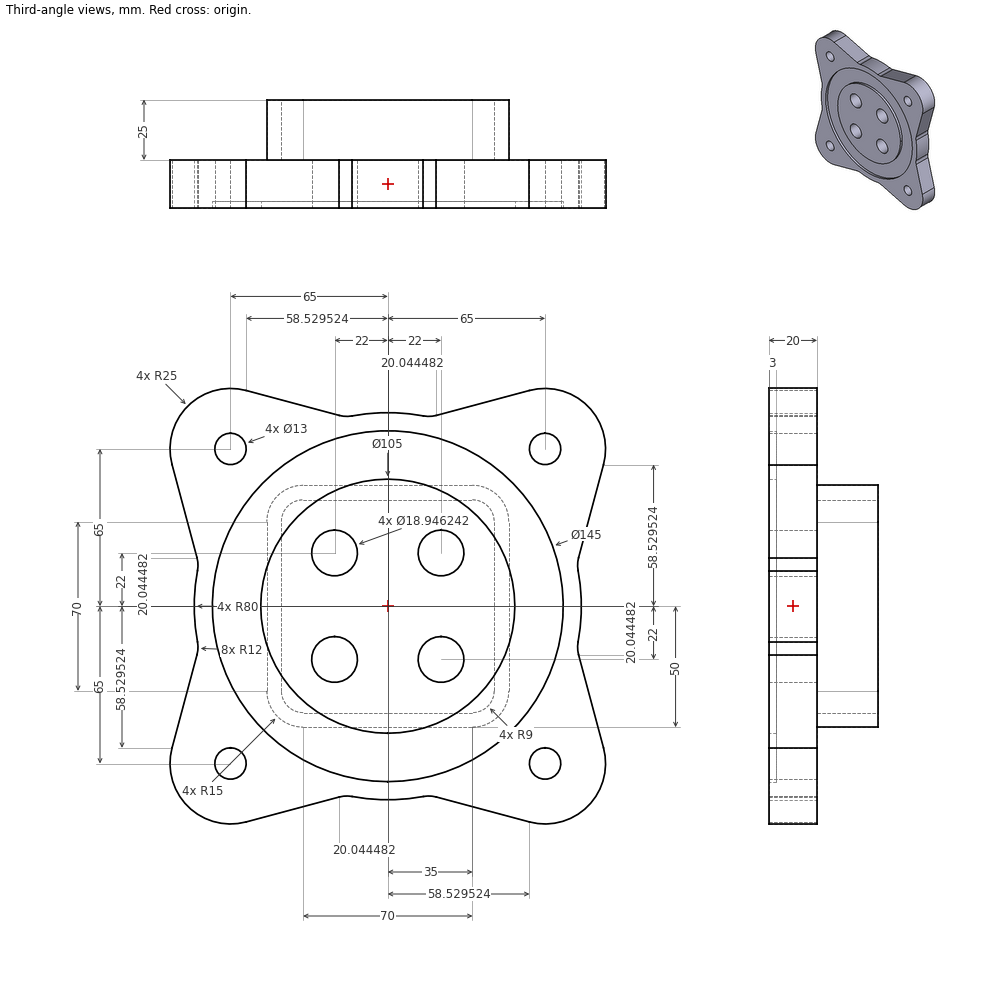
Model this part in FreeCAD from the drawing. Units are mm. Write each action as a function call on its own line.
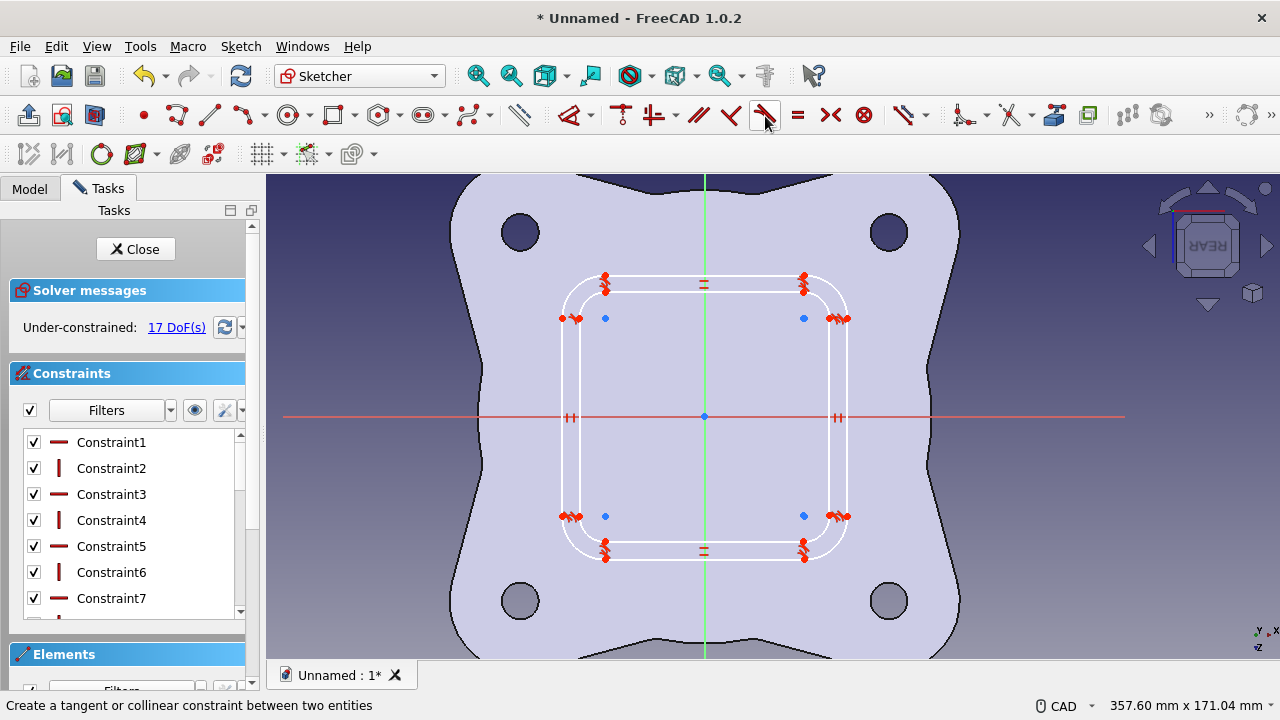
click(580, 457)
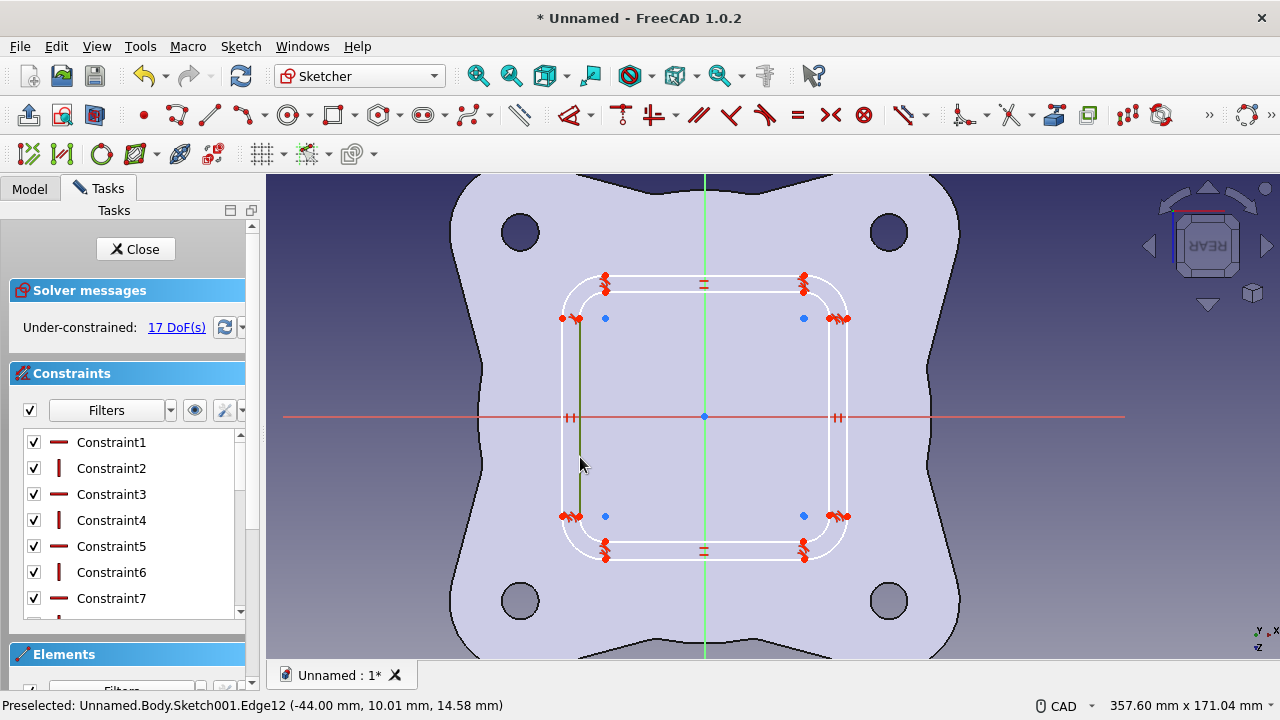
click(594, 295)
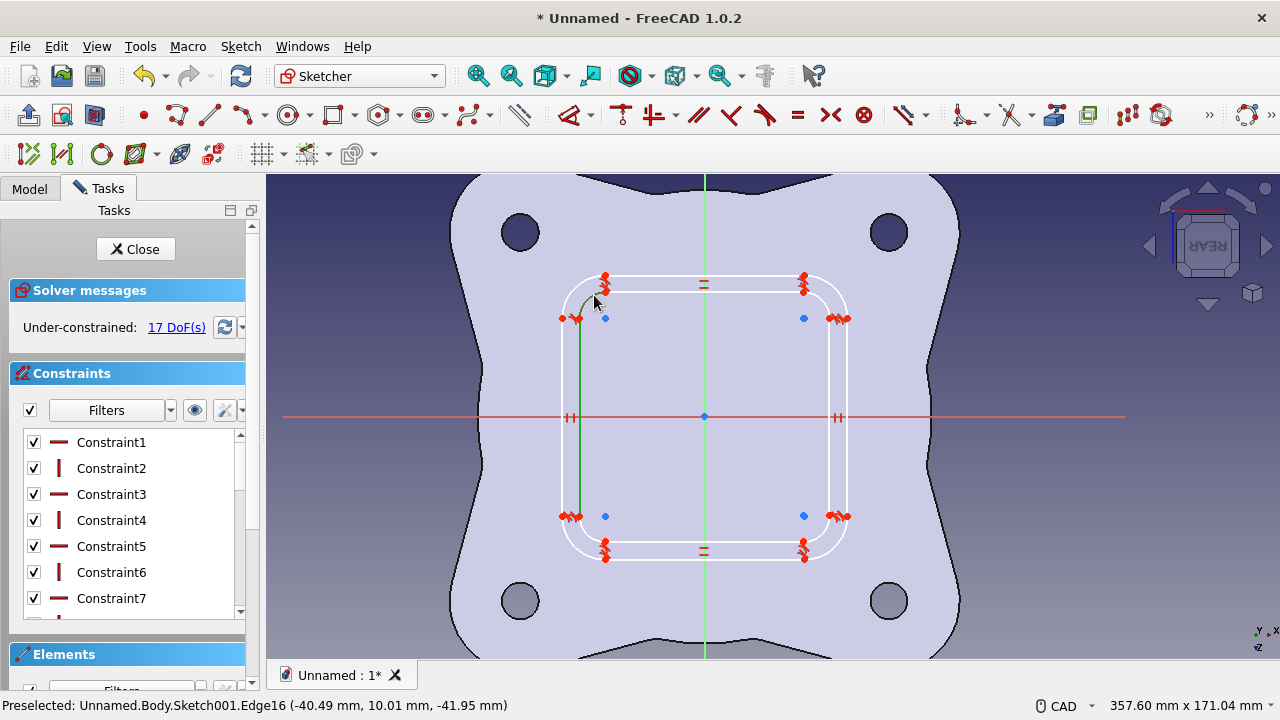
click(765, 116)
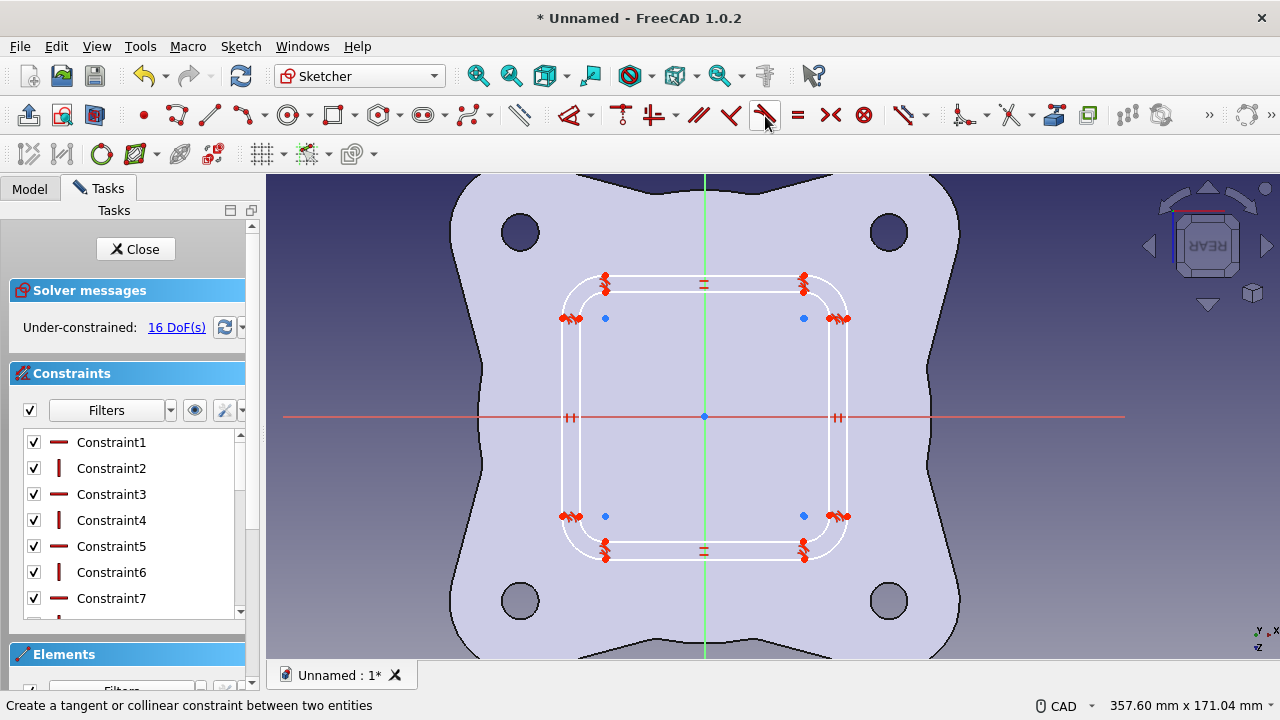
click(843, 299)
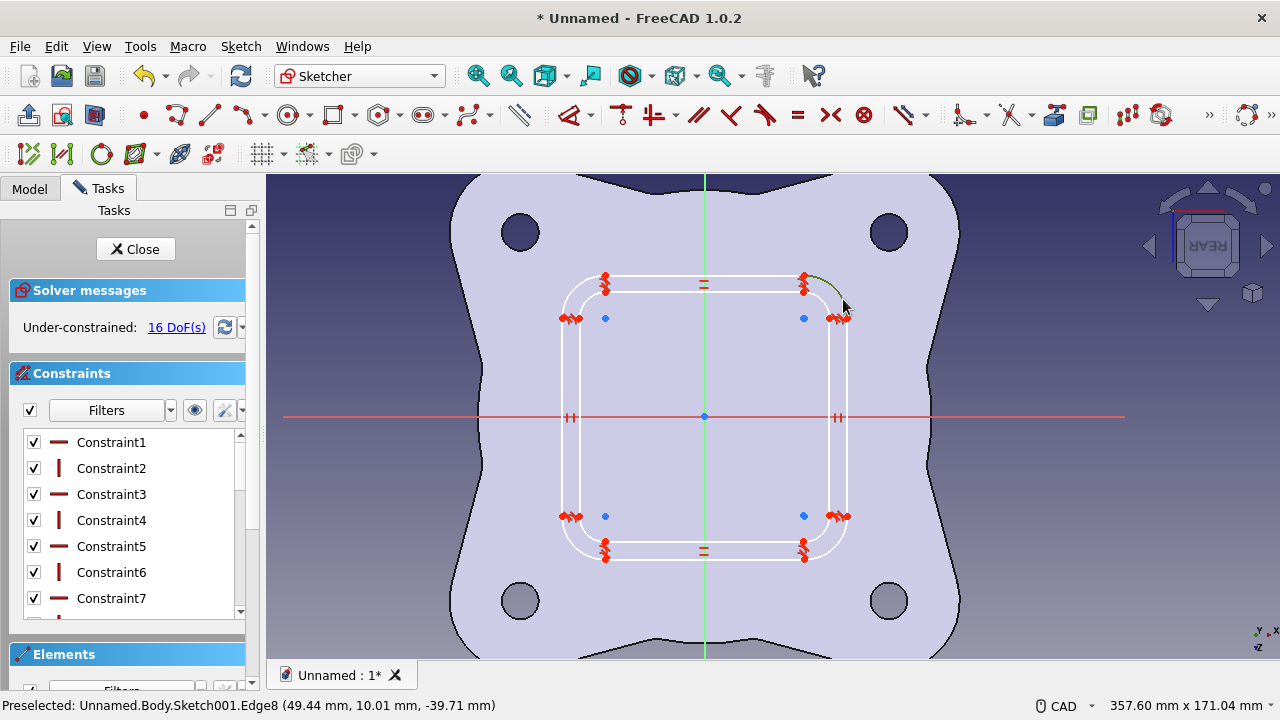
click(827, 307)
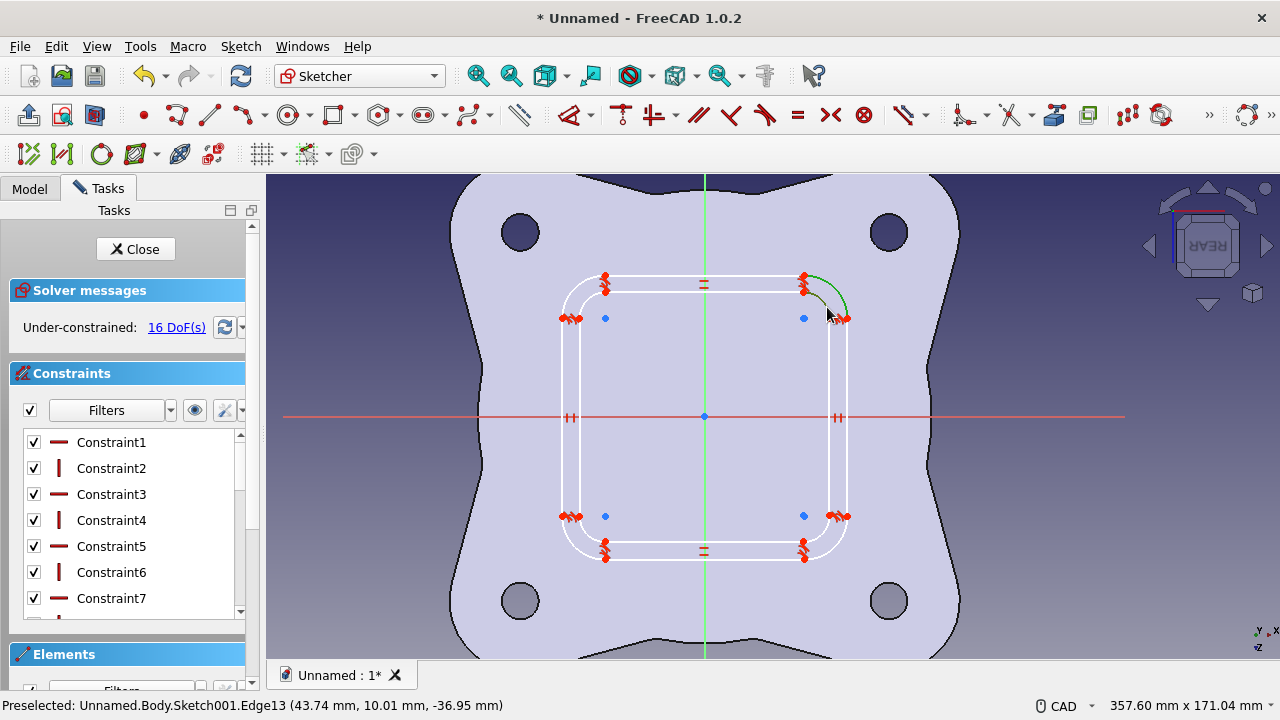
click(621, 116)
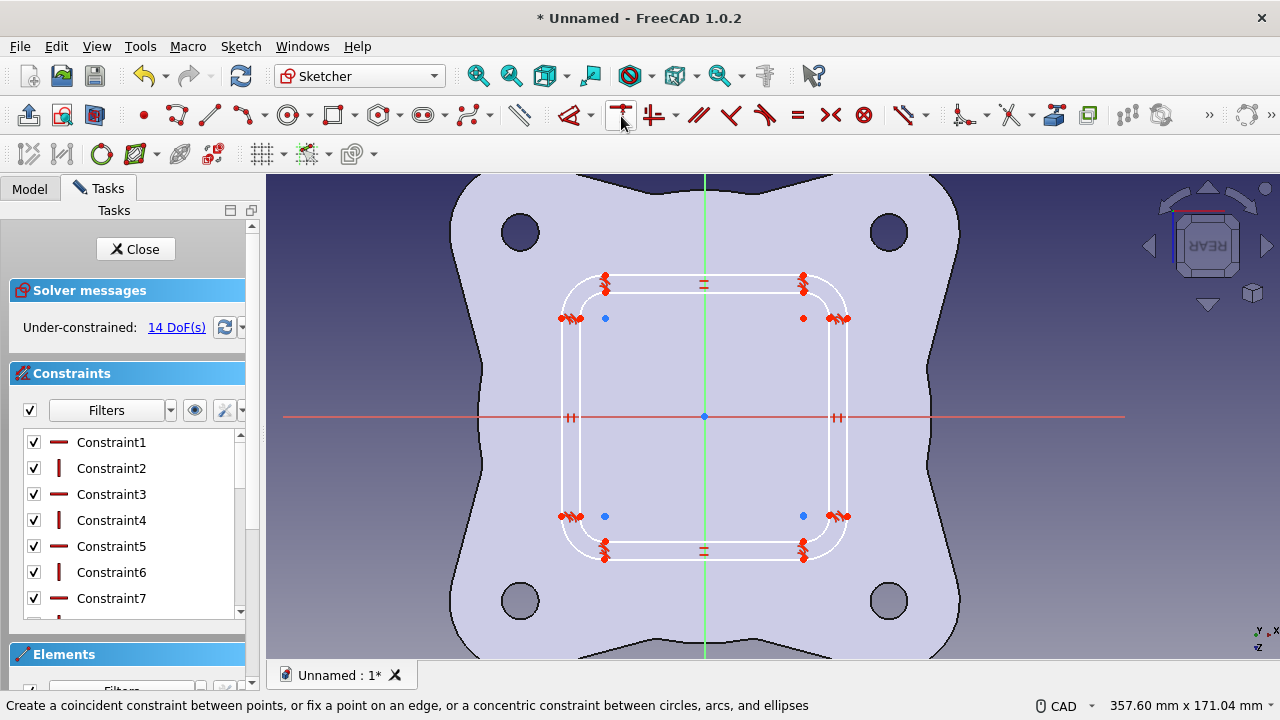
click(824, 555)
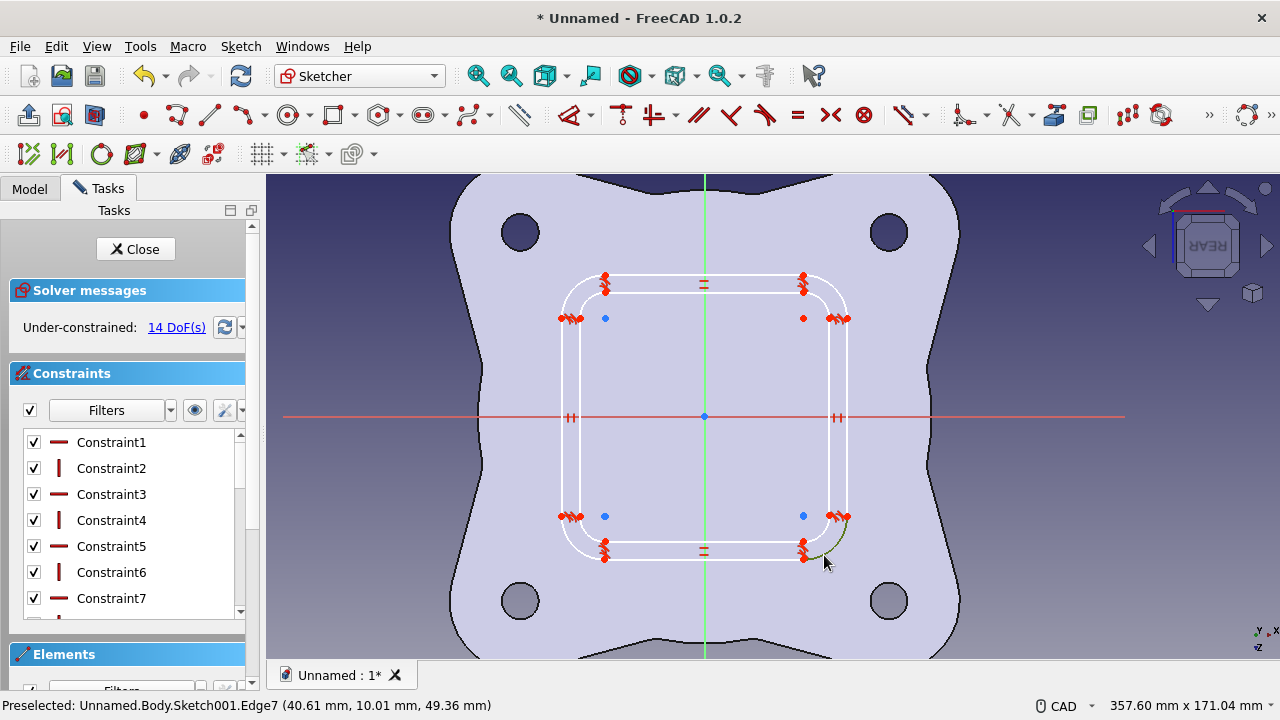
click(815, 539)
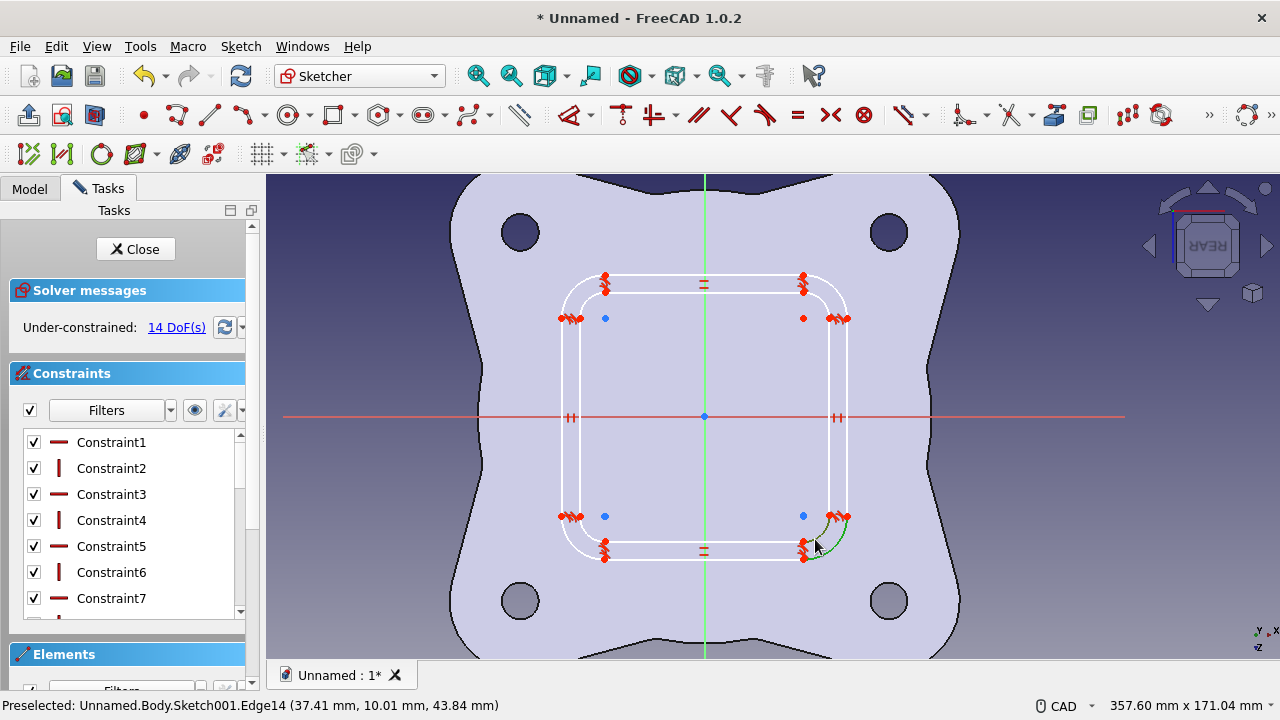
click(621, 116)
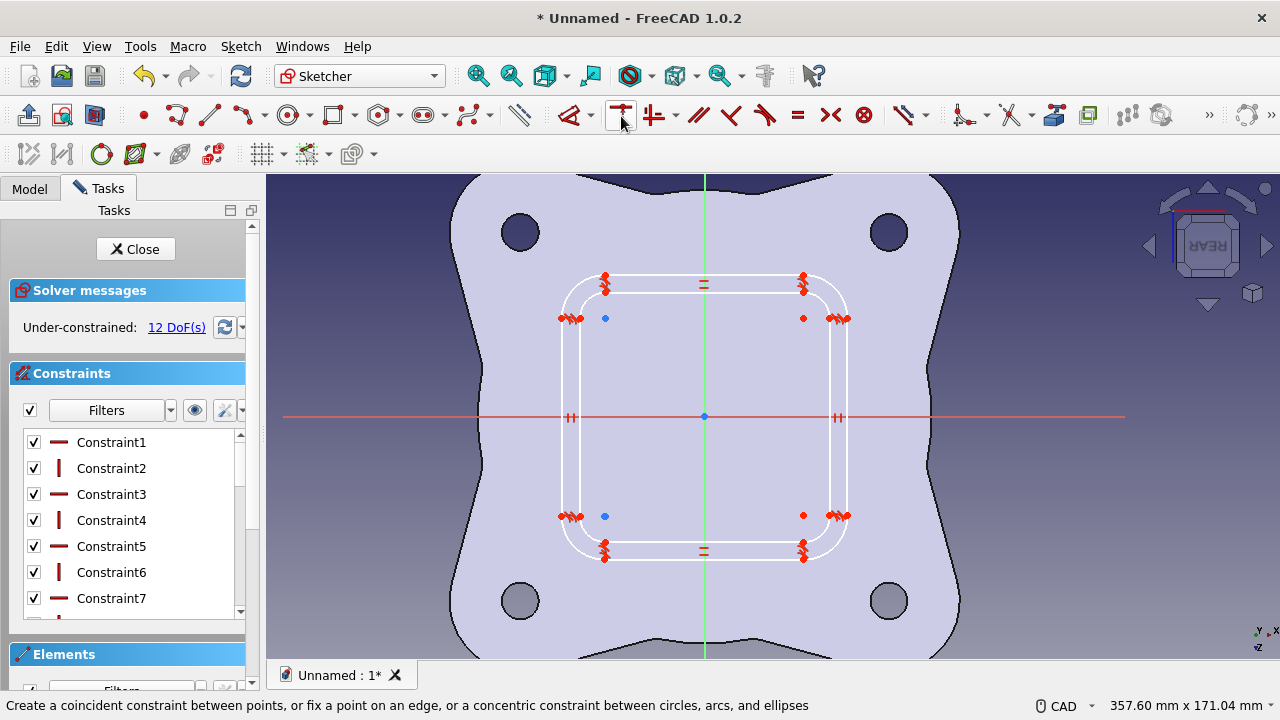
click(567, 536)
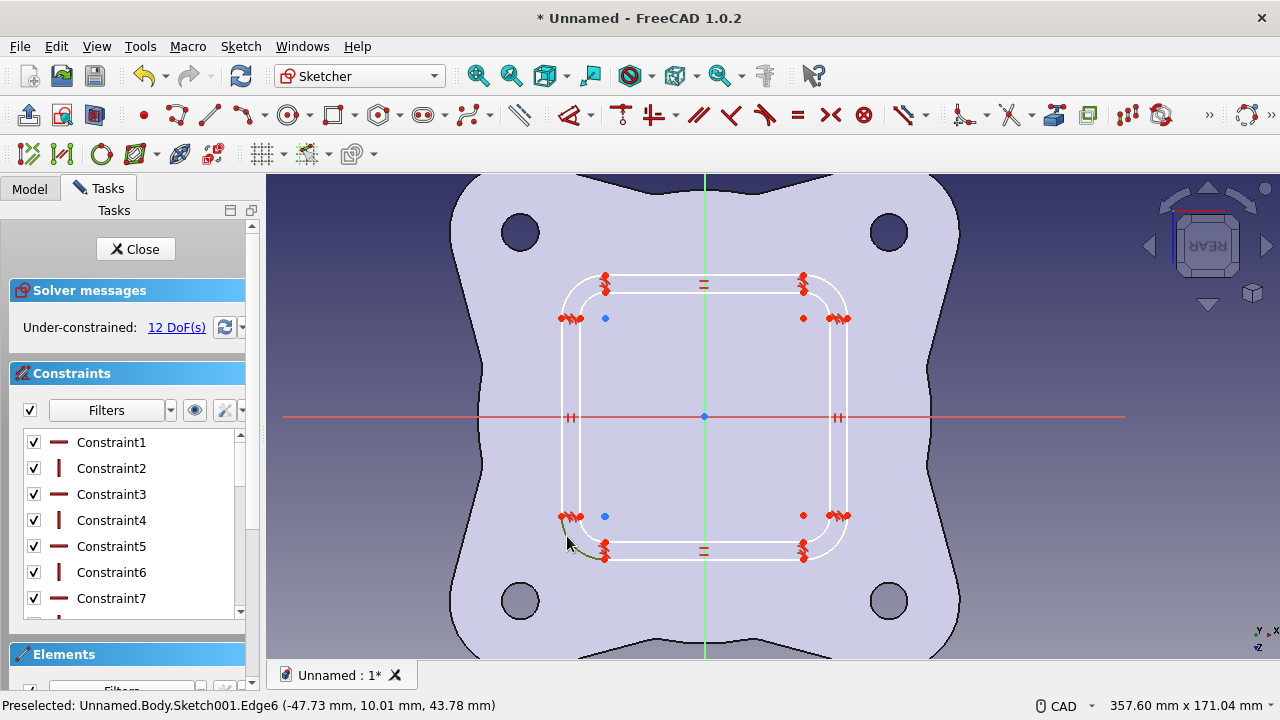
click(583, 528)